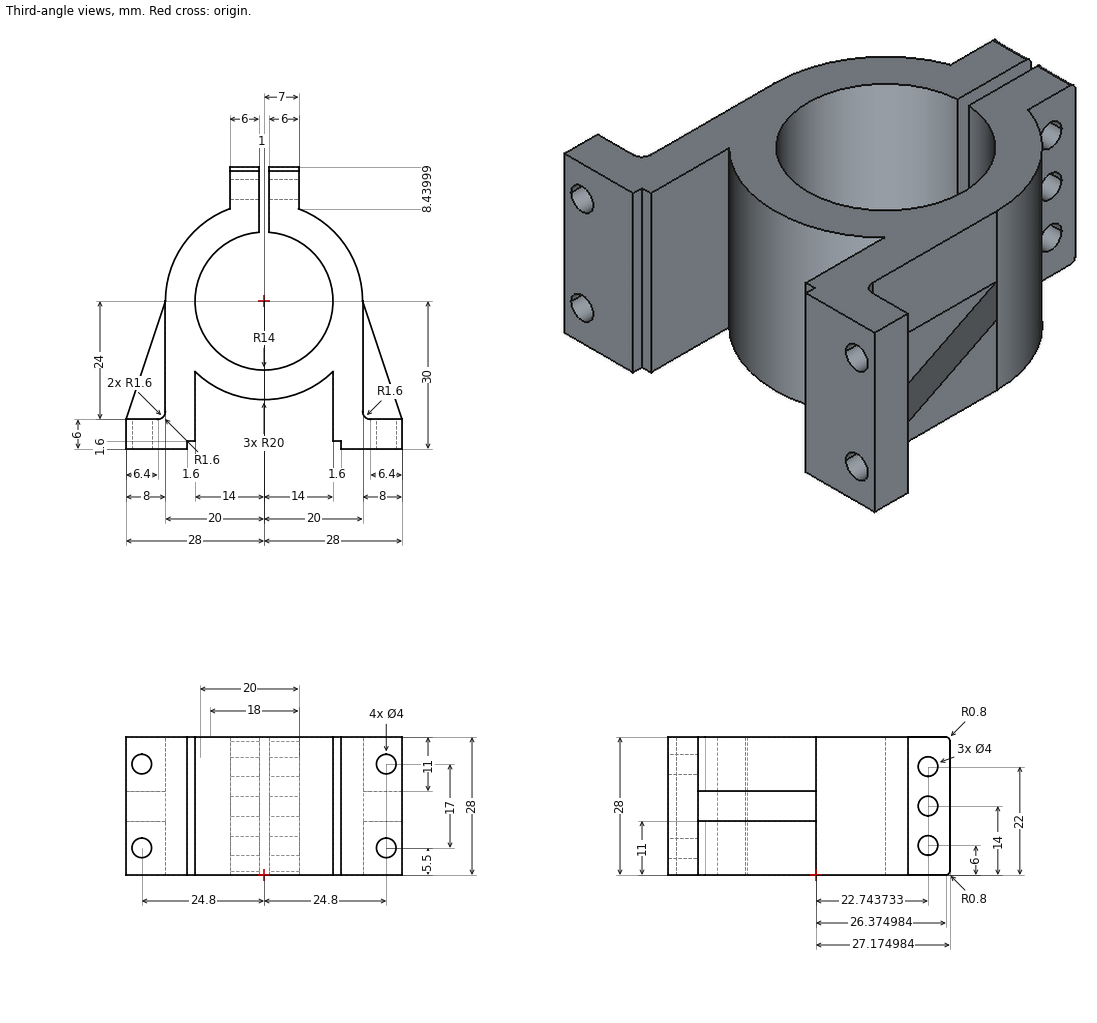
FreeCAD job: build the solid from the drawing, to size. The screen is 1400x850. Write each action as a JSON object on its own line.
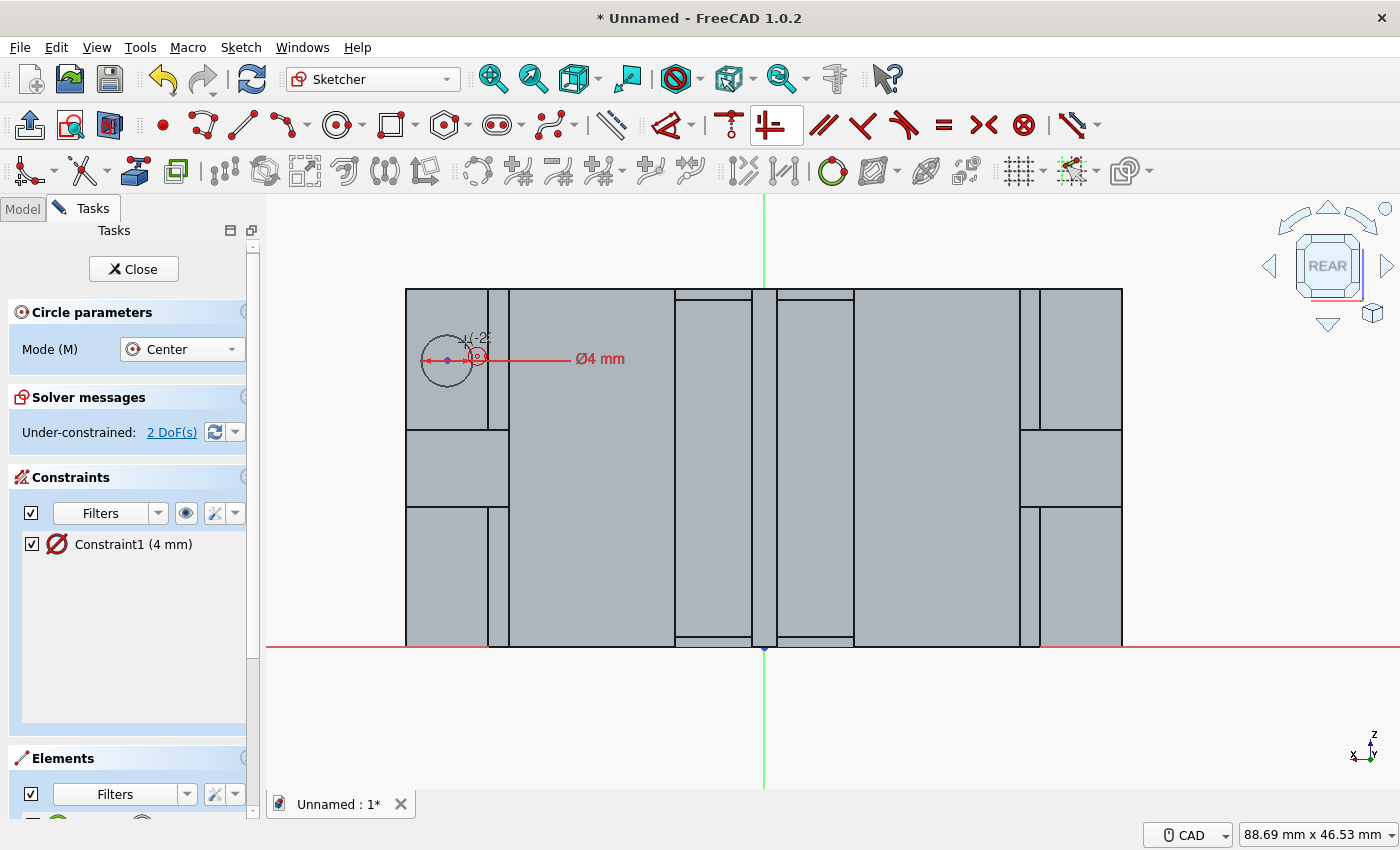
{"action": "left_click", "coordinate": [447, 577]}
{"action": "mouse_move", "coordinate": [465, 559]}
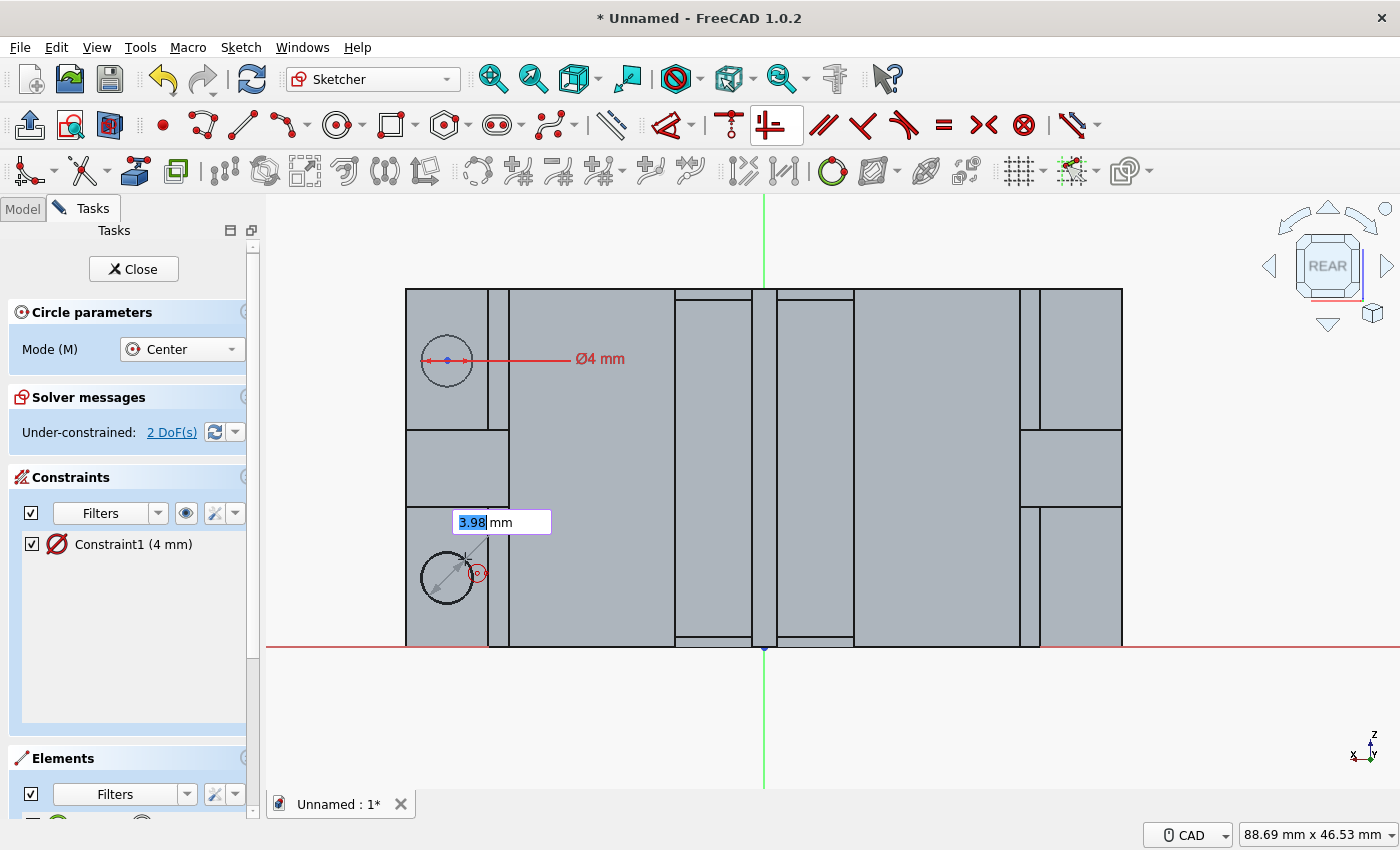
{"action": "type", "text": "4"}
{"action": "key", "text": "Return"}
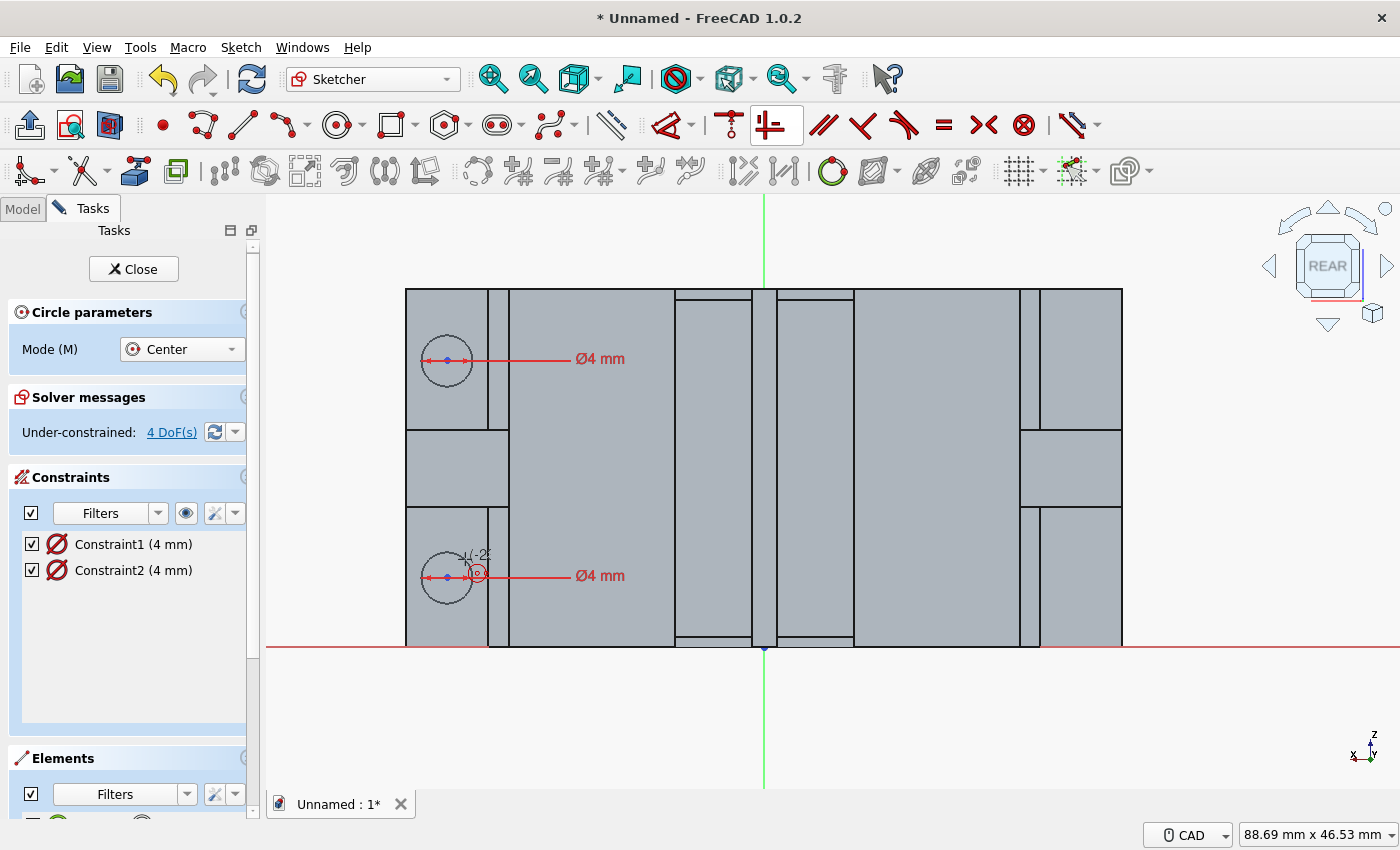
{"action": "left_click", "coordinate": [1081, 577]}
{"action": "mouse_move", "coordinate": [1099, 559]}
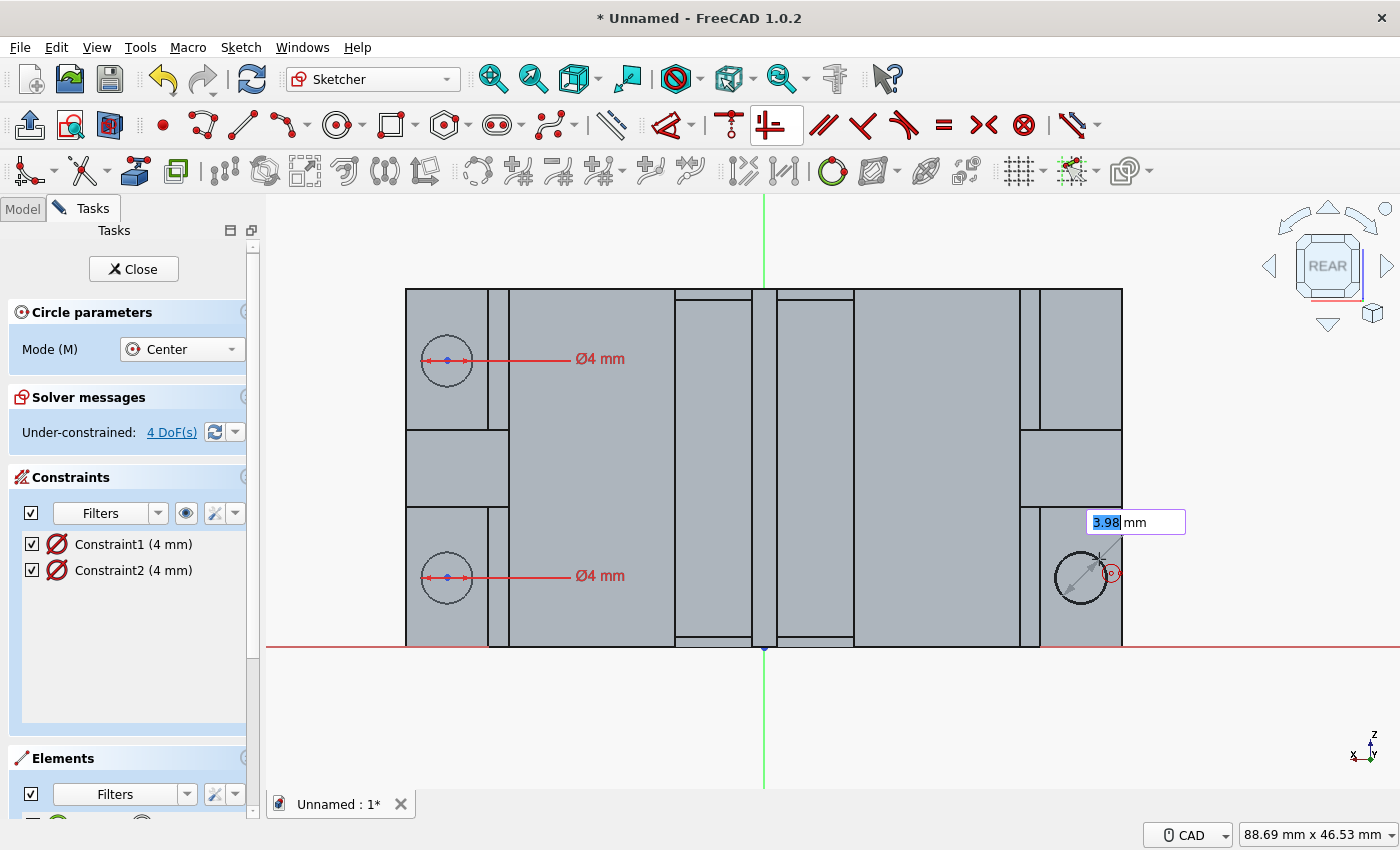
{"action": "type", "text": "4"}
{"action": "key", "text": "Return"}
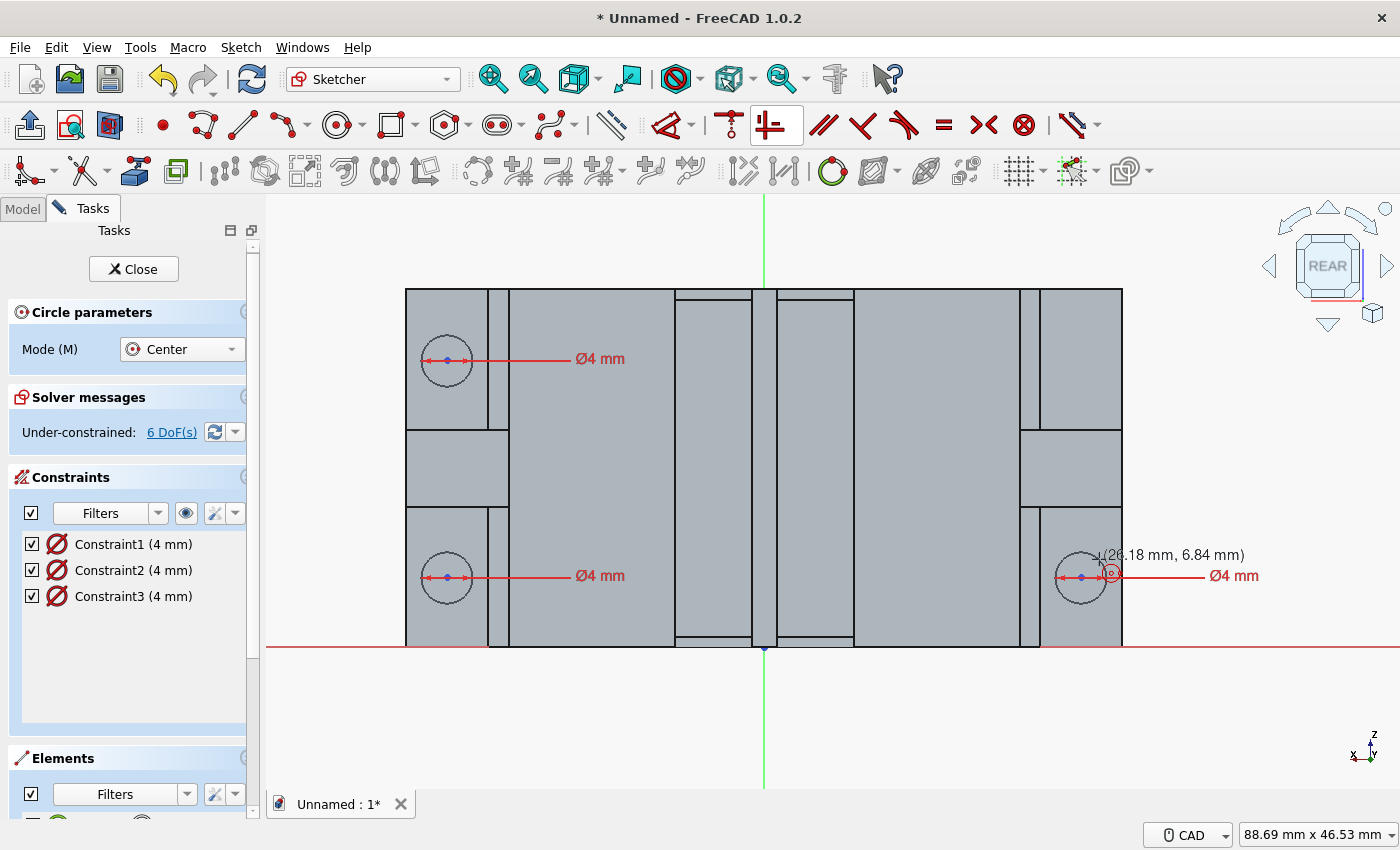
{"action": "left_click", "coordinate": [1081, 360]}
{"action": "mouse_move", "coordinate": [1099, 342]}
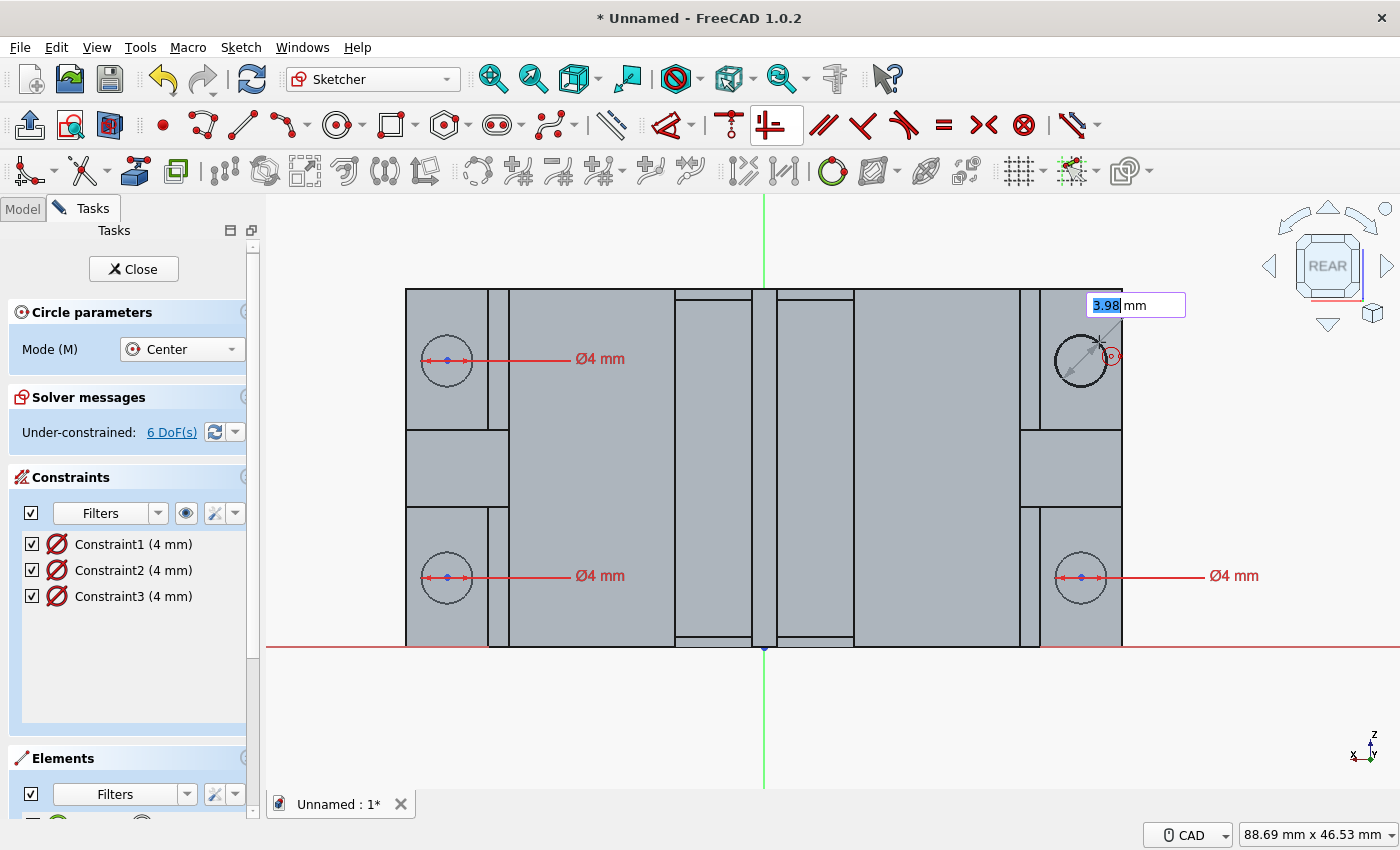
{"action": "type", "text": "4"}
{"action": "key", "text": "Return"}
{"action": "key", "text": "Escape"}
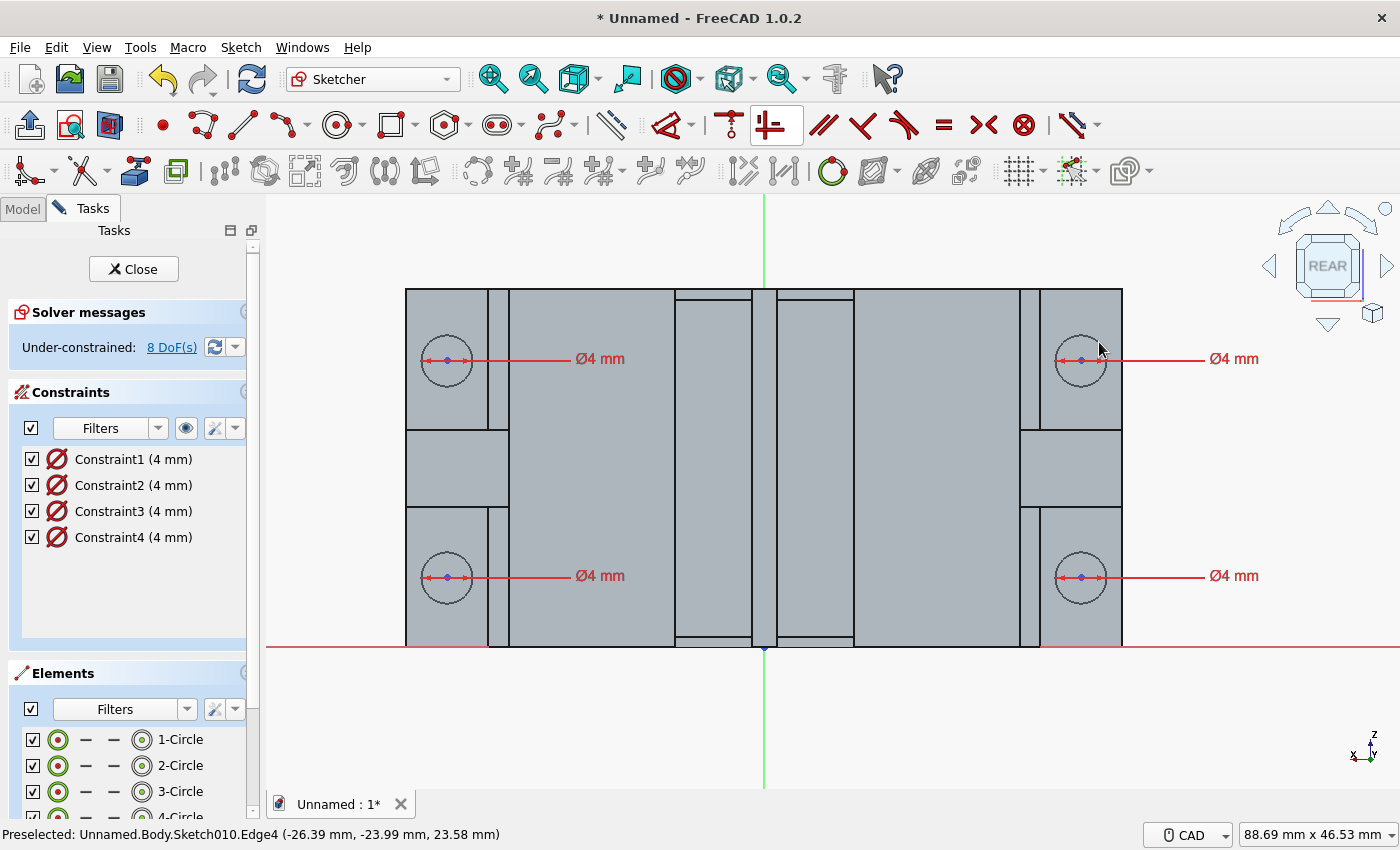
{"action": "left_click", "coordinate": [447, 361]}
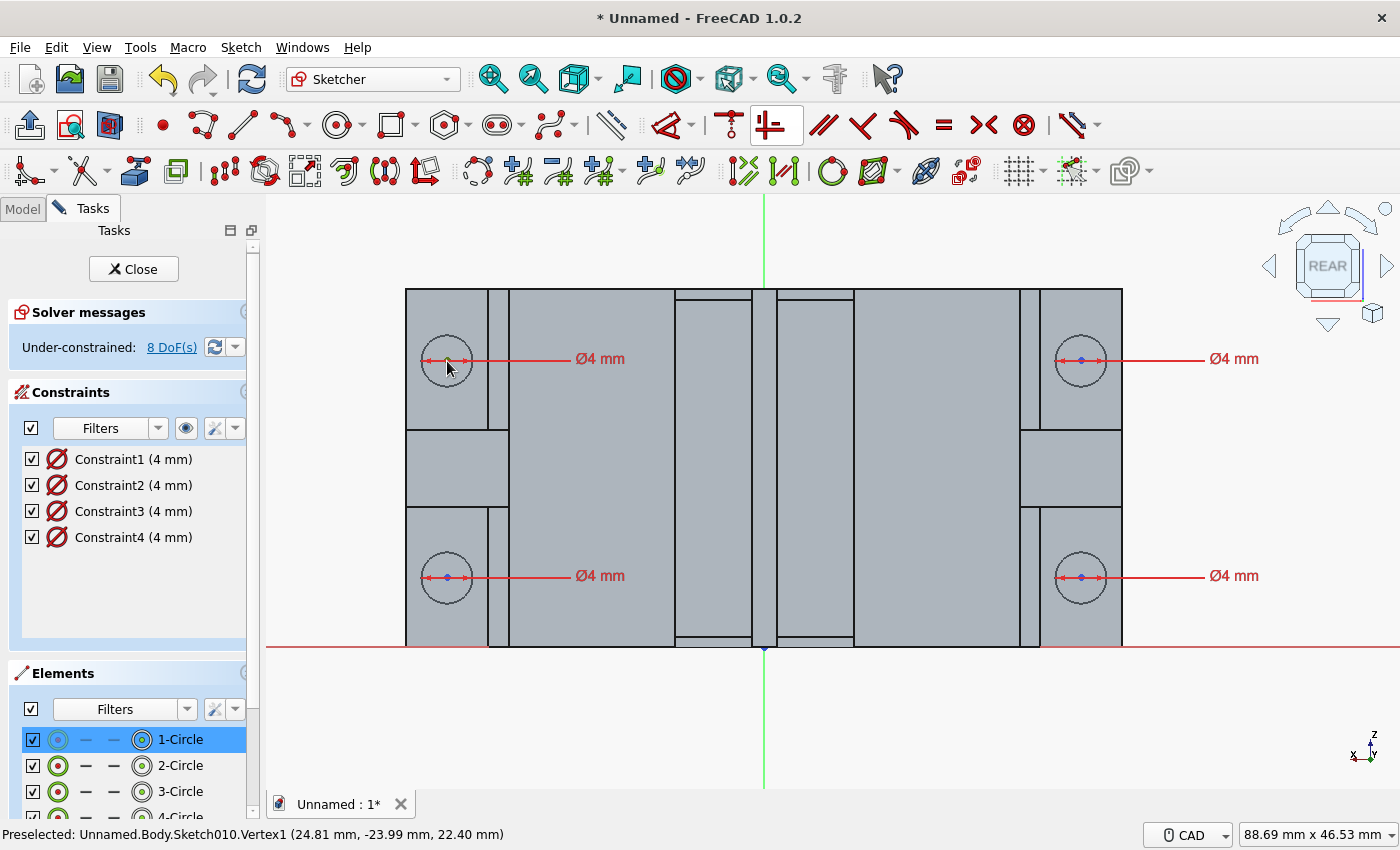
{"action": "left_click", "coordinate": [447, 578]}